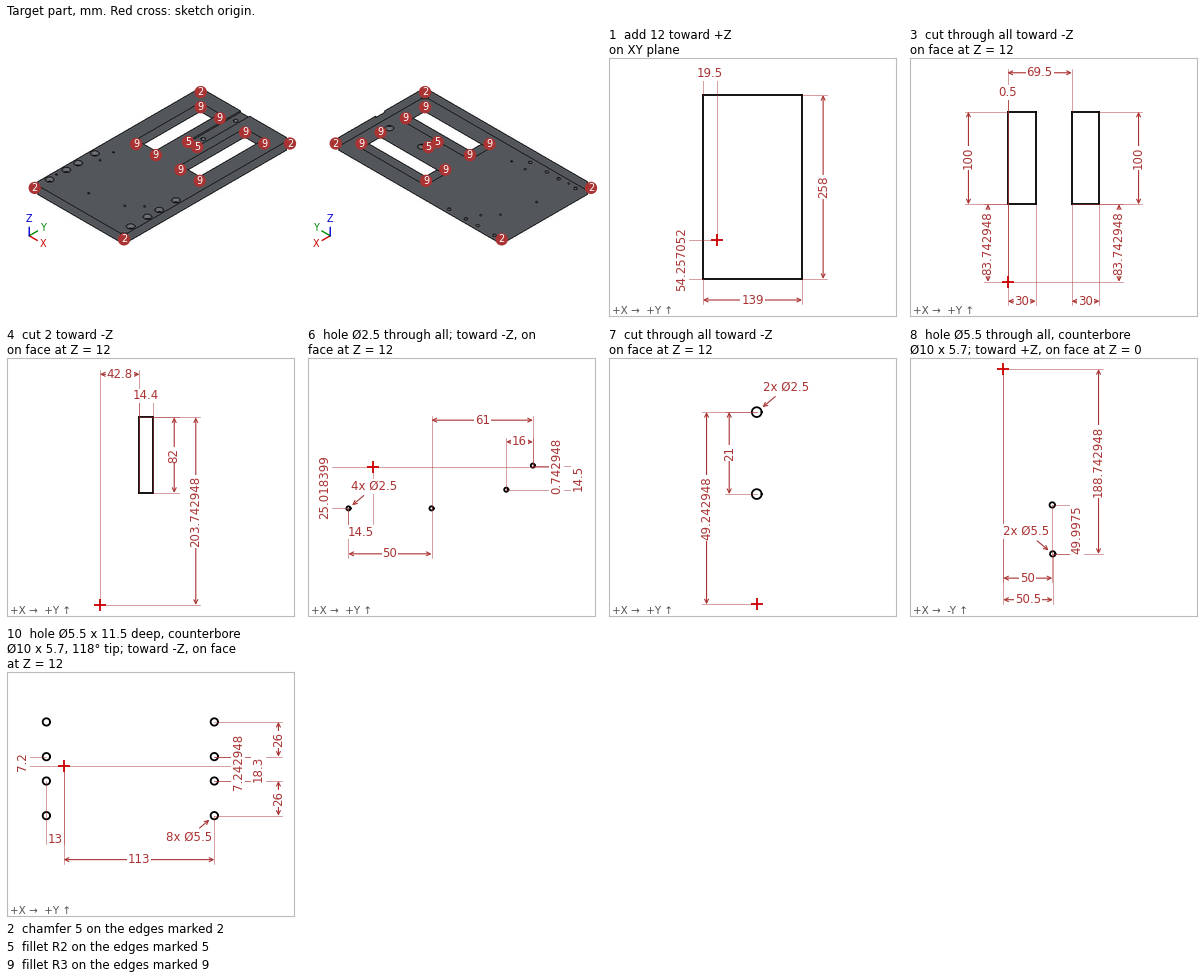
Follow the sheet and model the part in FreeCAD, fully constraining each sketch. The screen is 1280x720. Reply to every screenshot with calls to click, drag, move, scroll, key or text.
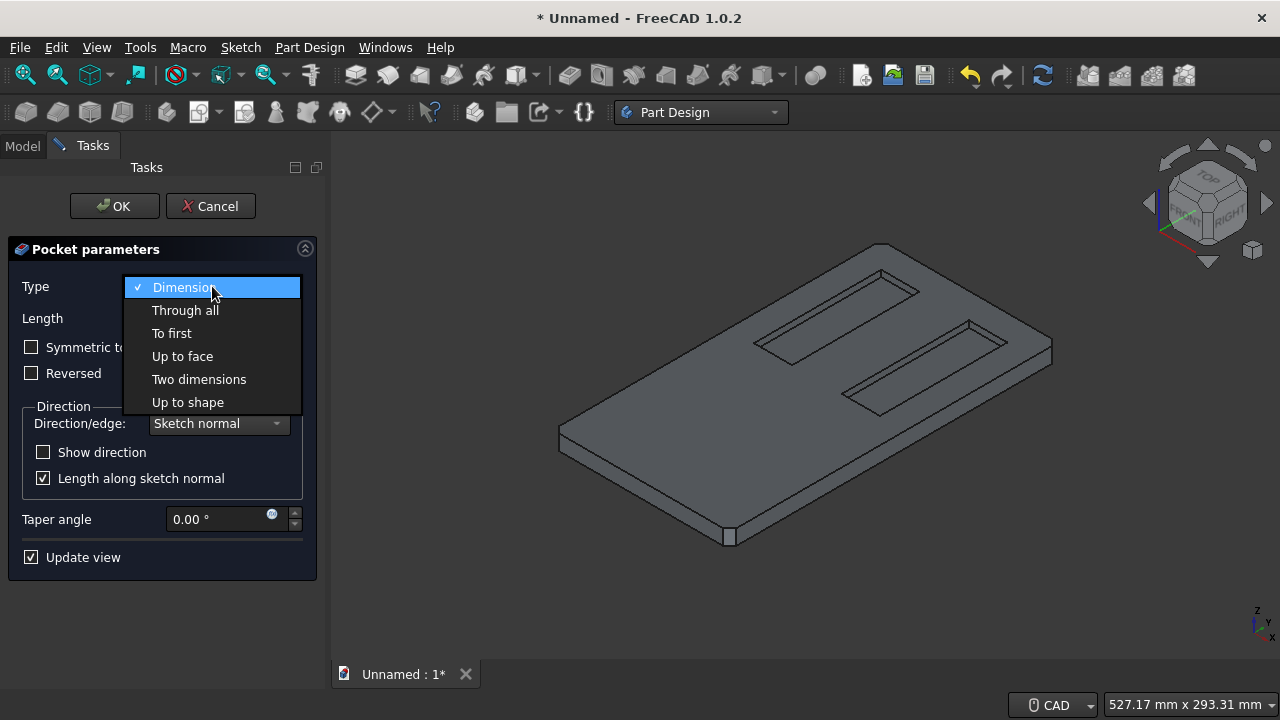
click(212, 310)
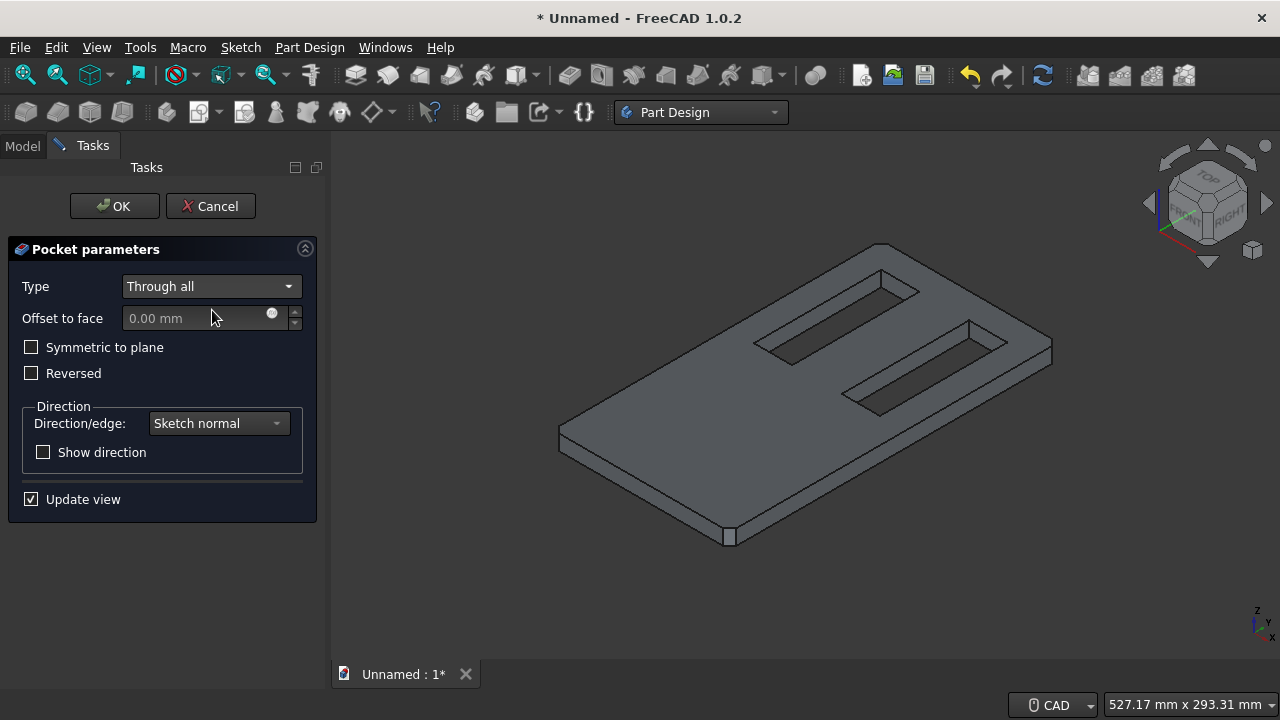
click(115, 206)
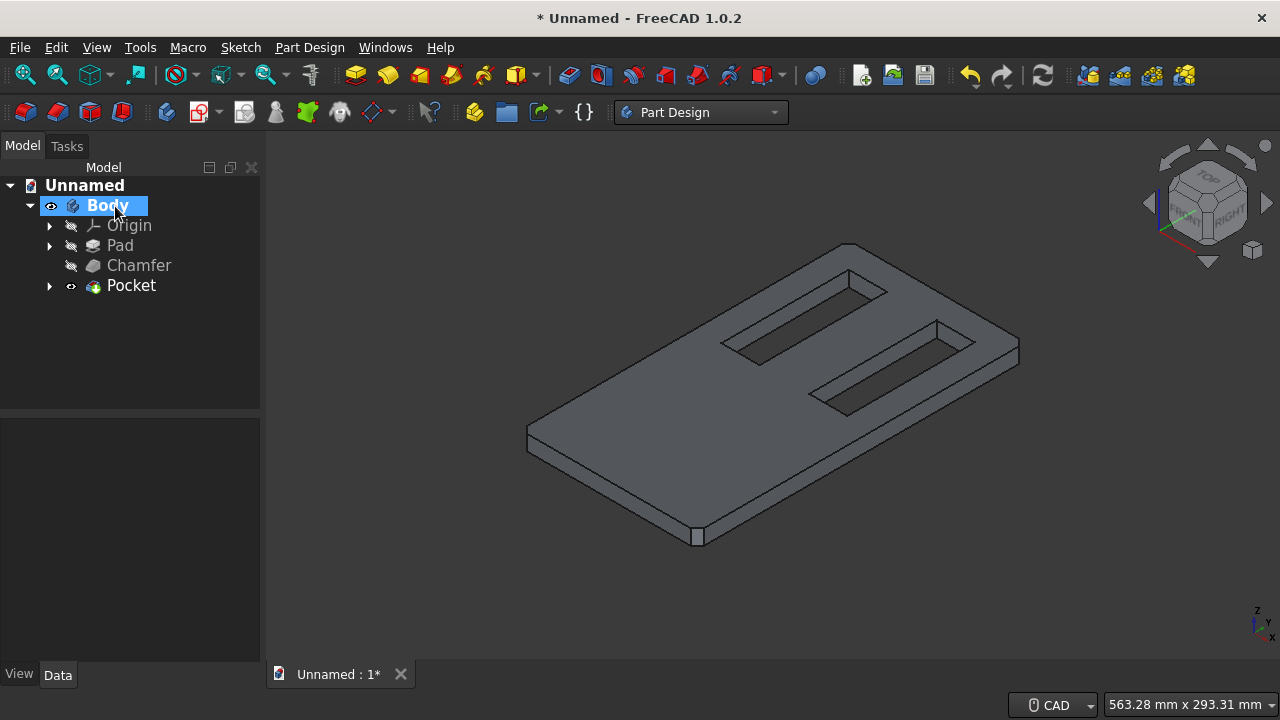
click(679, 439)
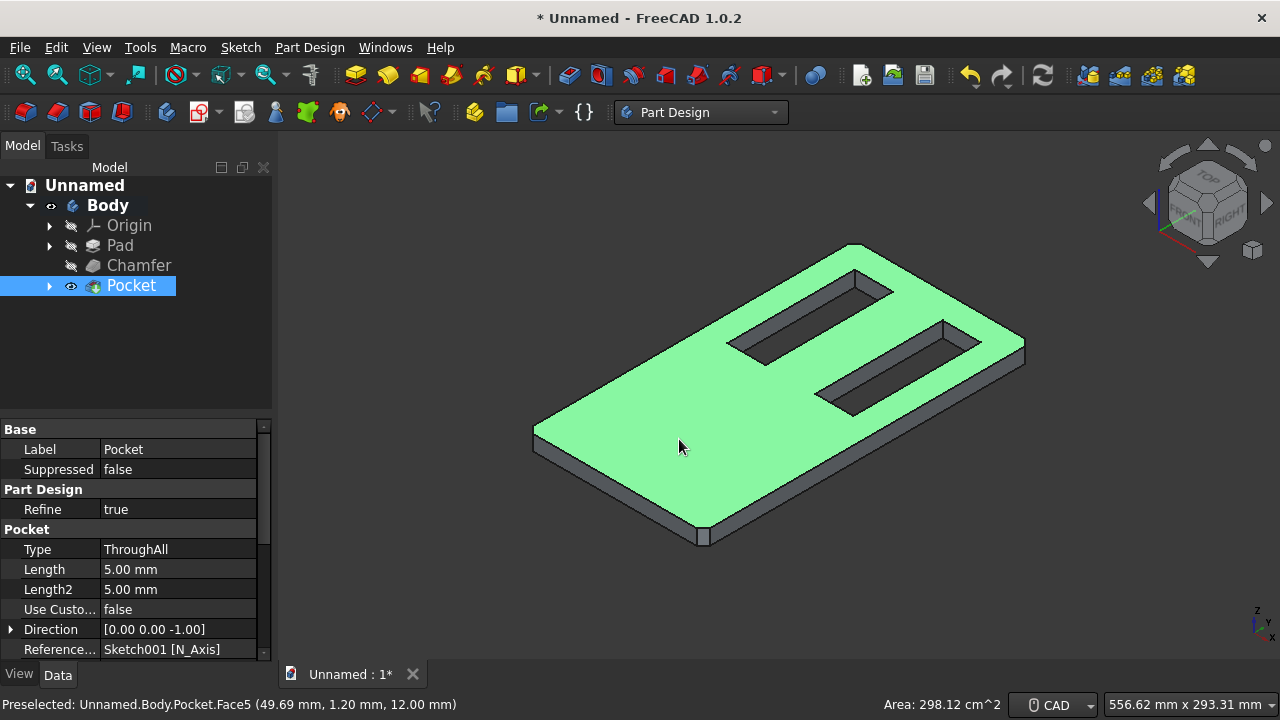
click(200, 112)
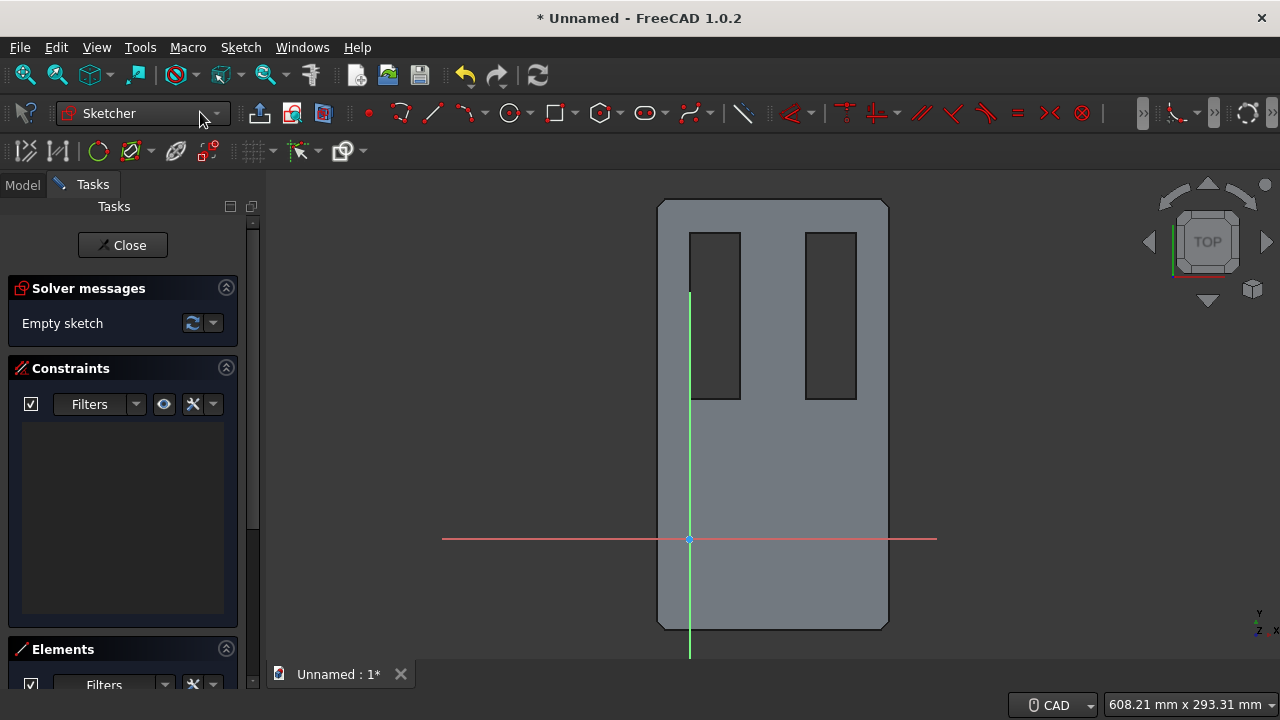
scroll(556, 619, down, 1)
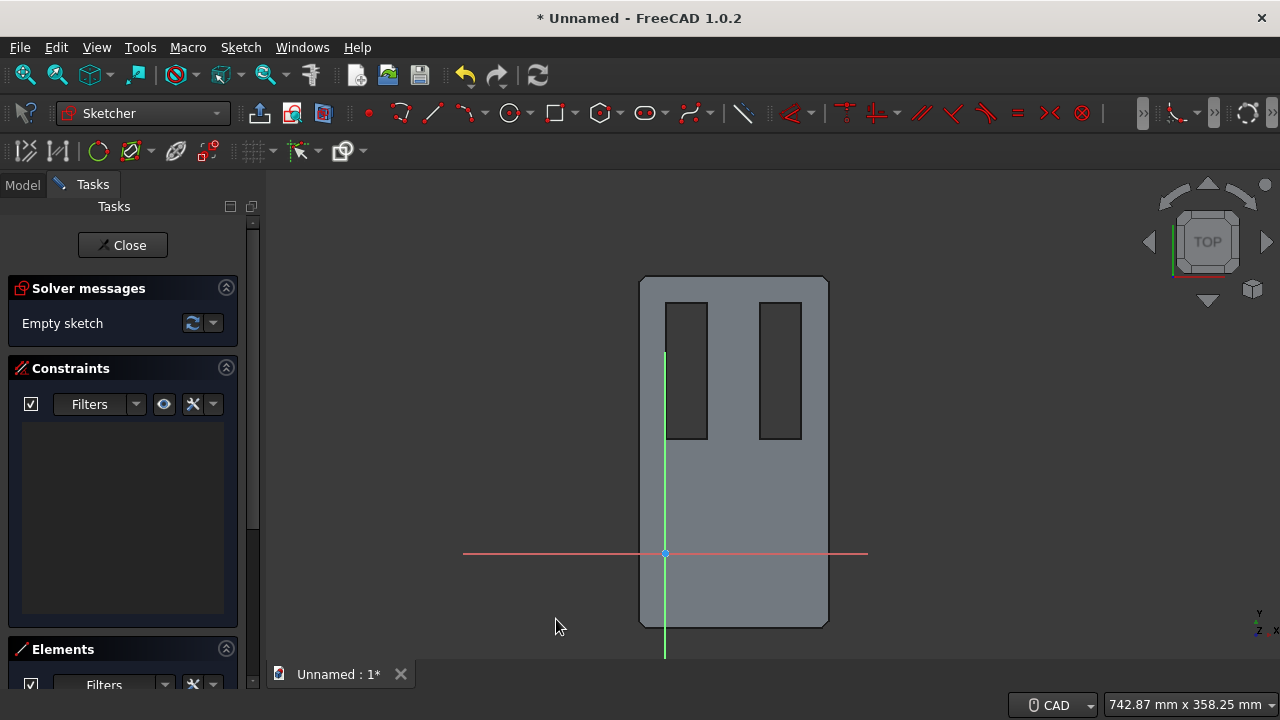
key(g)
key(r)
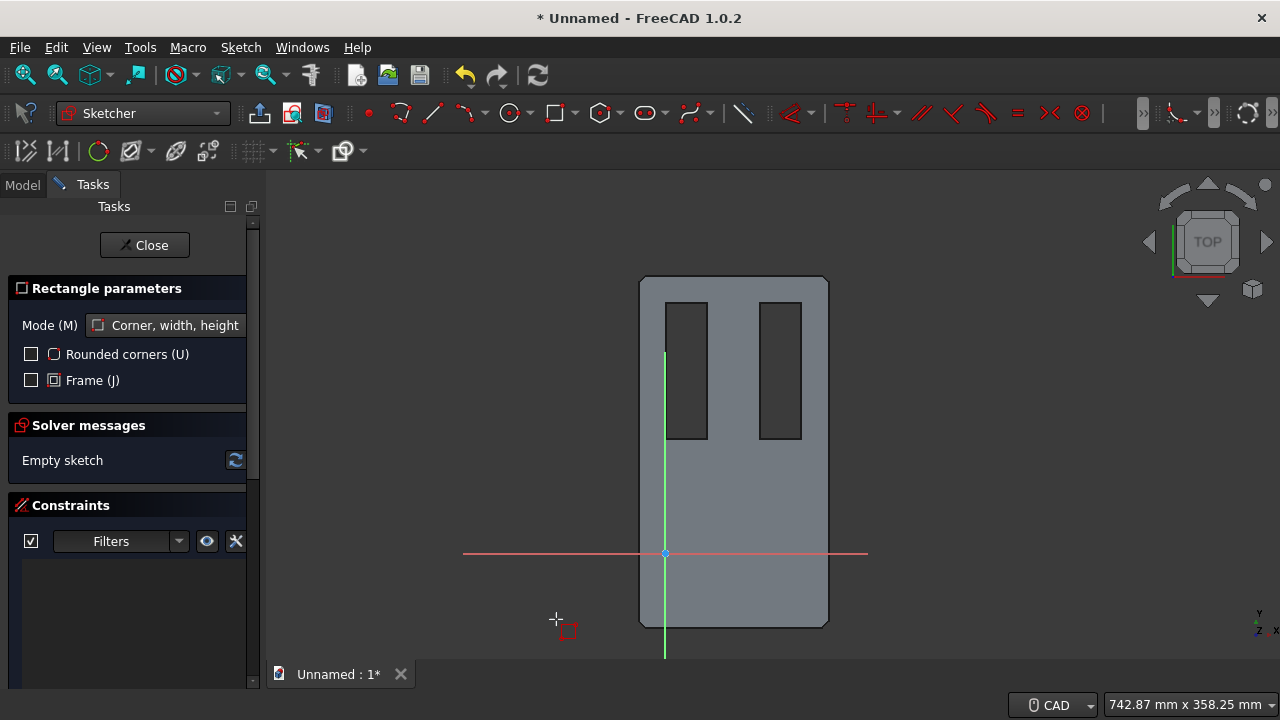
click(724, 276)
move(744, 388)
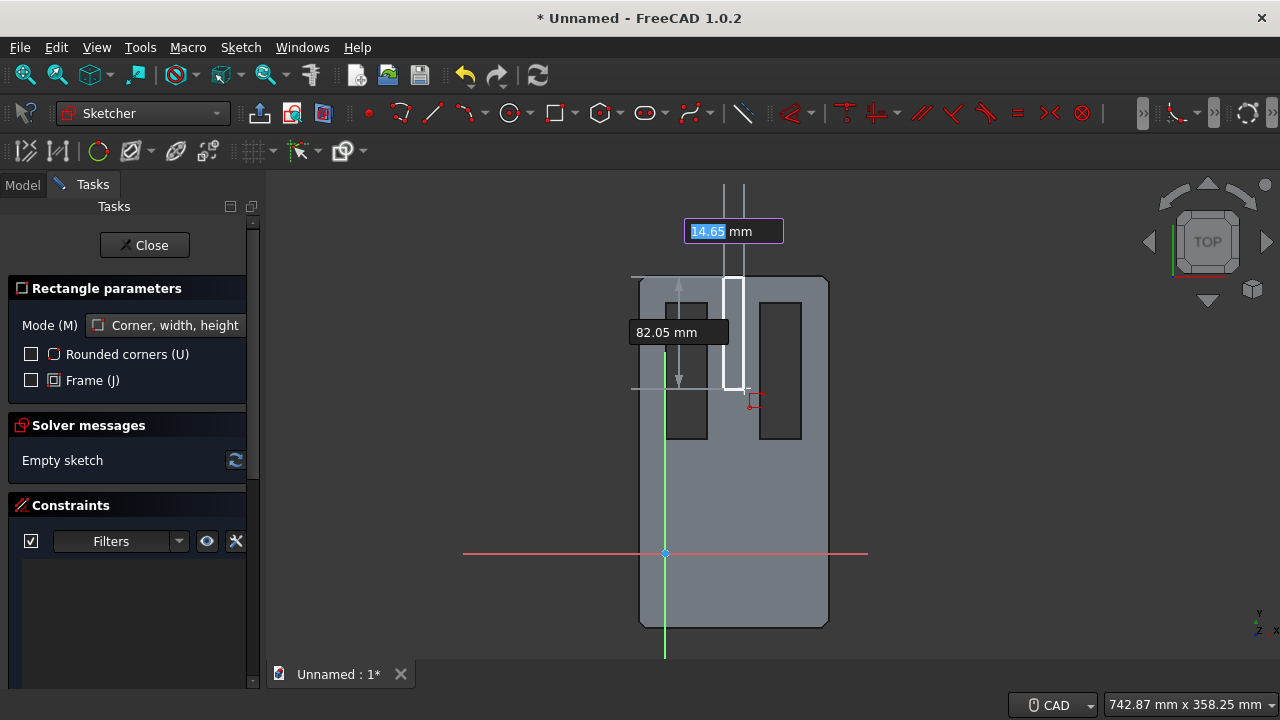
text(14.4)
key(Tab)
text(82)
key(Return)
key(Escape)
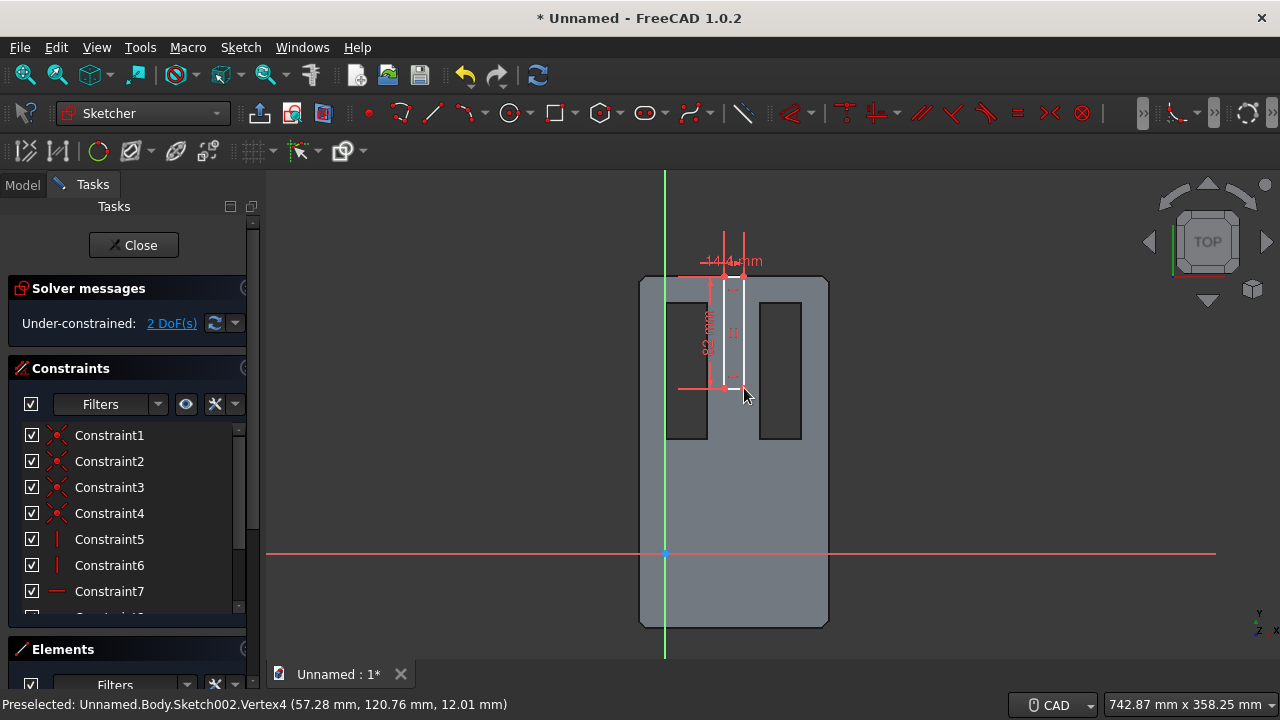
key(d)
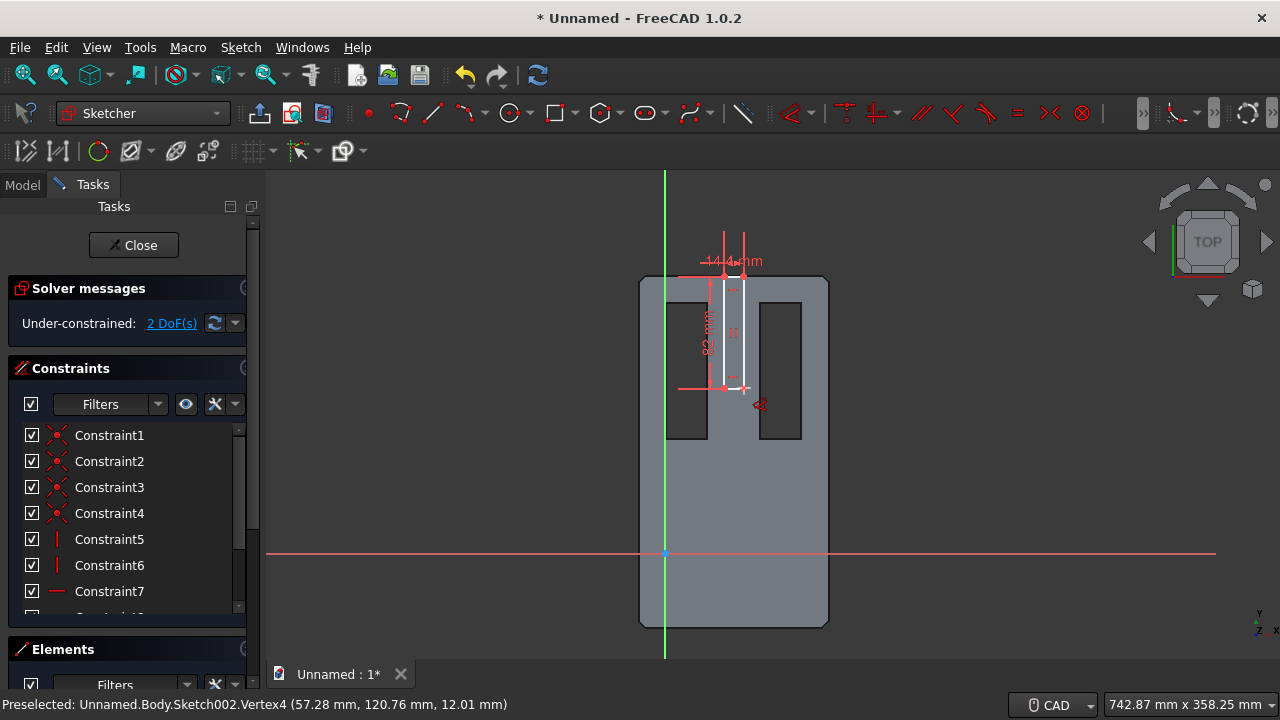
click(724, 277)
click(695, 588)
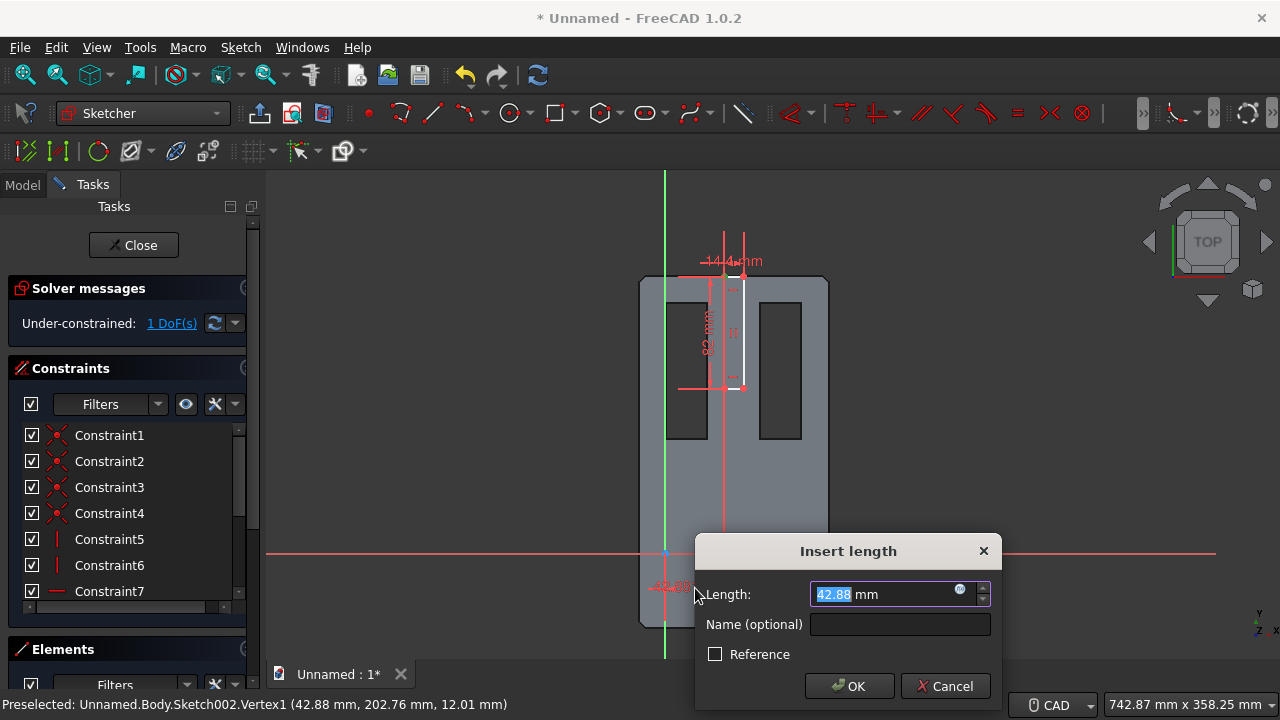
text(42.8)
key(Return)